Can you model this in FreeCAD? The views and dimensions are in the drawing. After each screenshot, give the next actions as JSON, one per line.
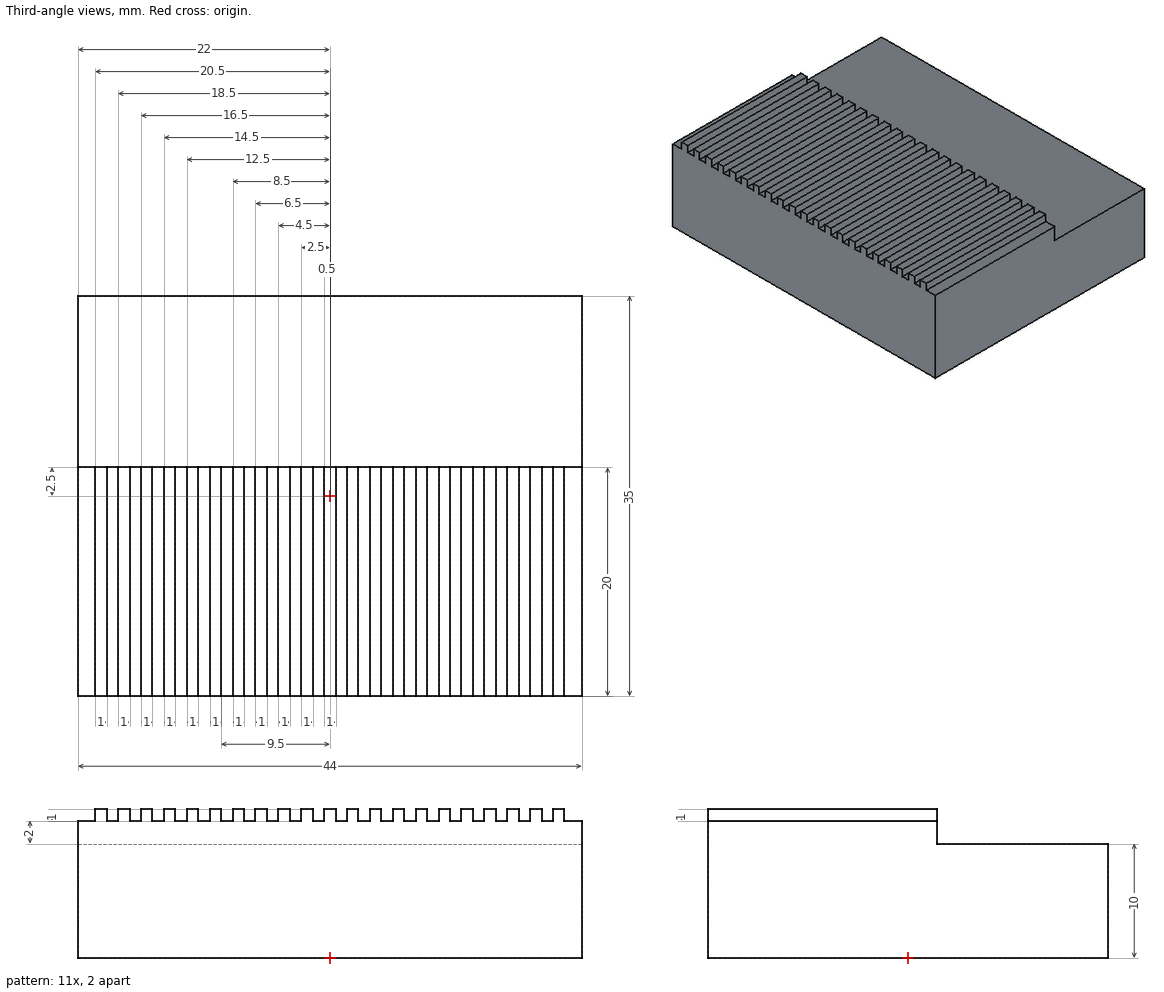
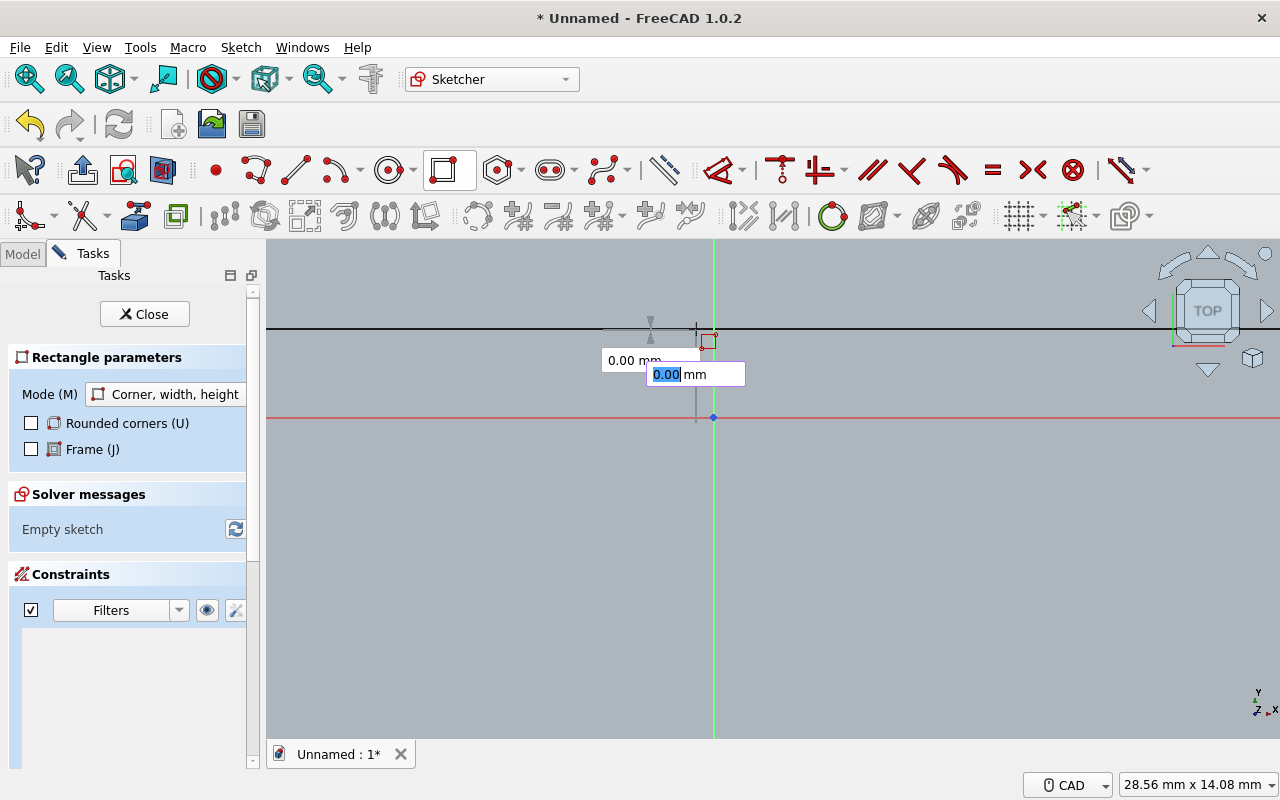
{"action": "scroll", "coordinate": [697, 330], "scroll_direction": "down", "scroll_amount": 4}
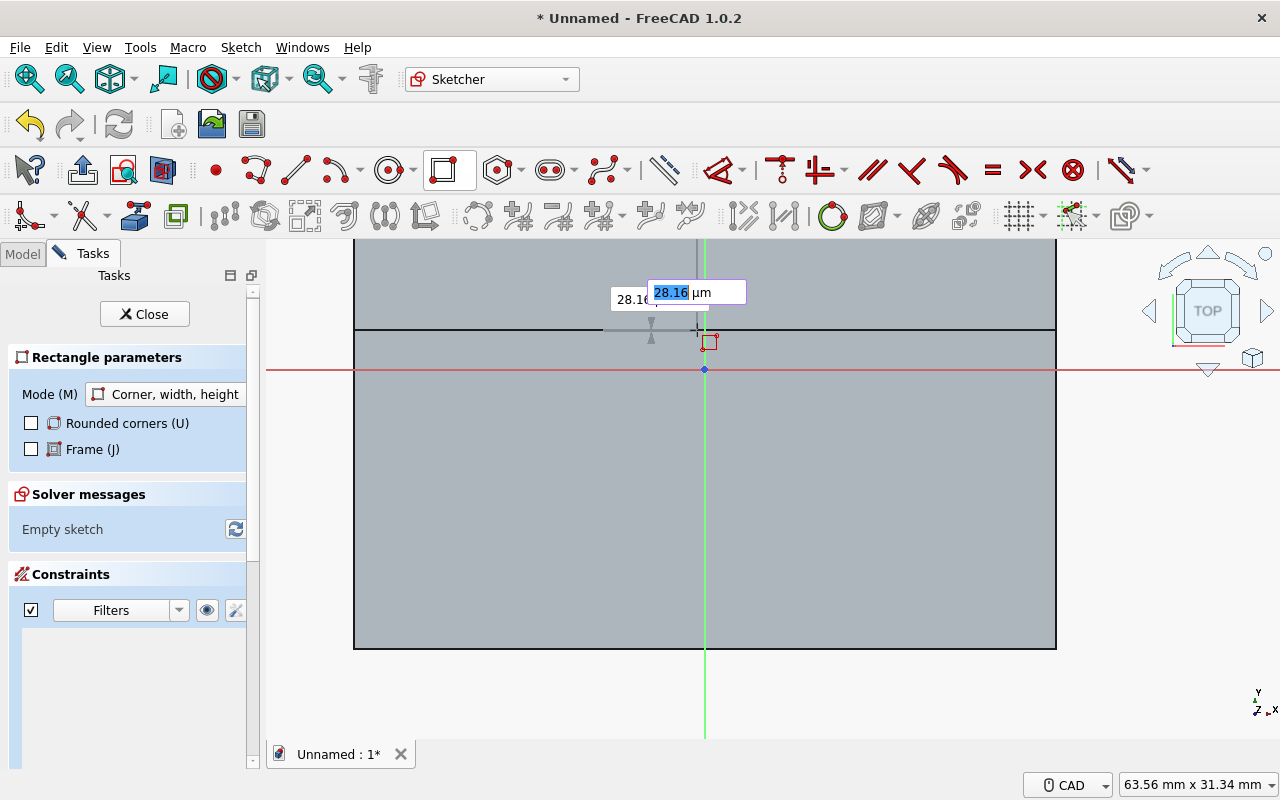
{"action": "scroll", "coordinate": [713, 649], "scroll_direction": "up", "scroll_amount": 4}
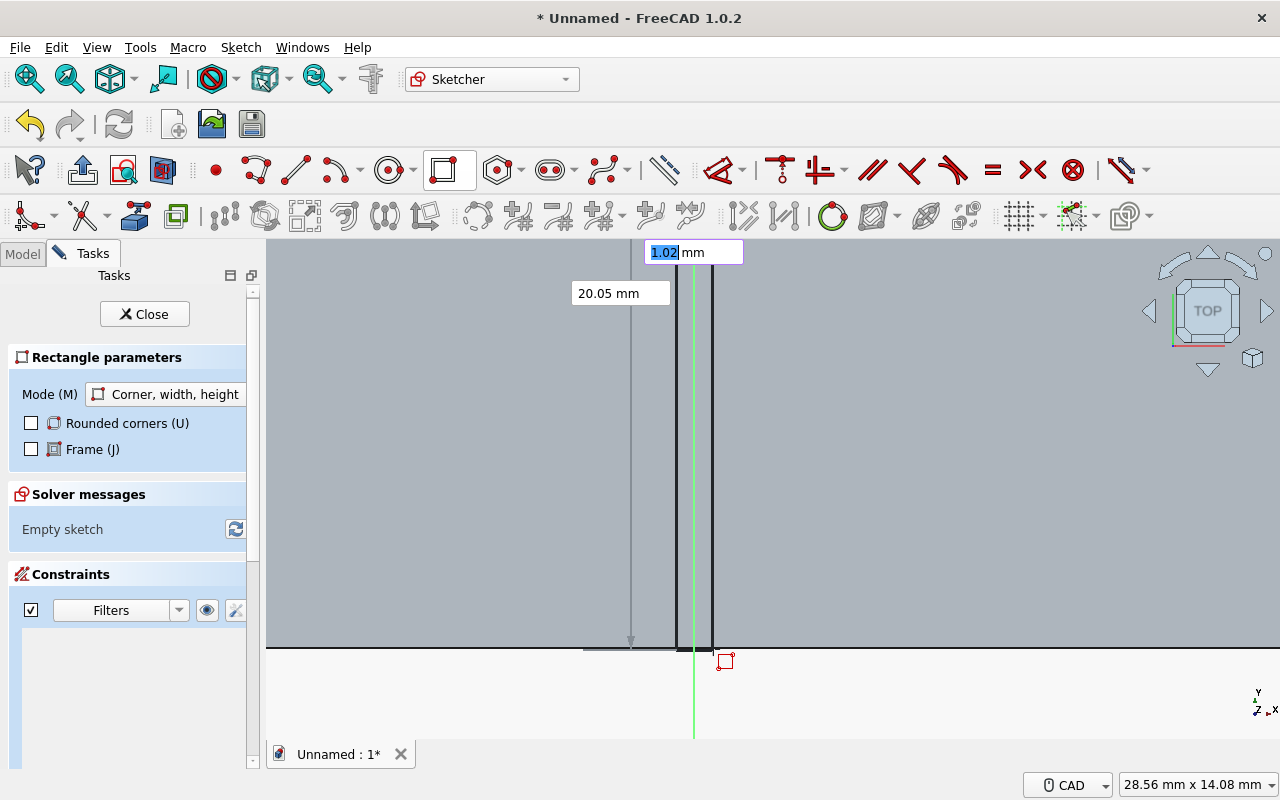
{"action": "left_click", "coordinate": [712, 648]}
{"action": "key", "text": "Escape"}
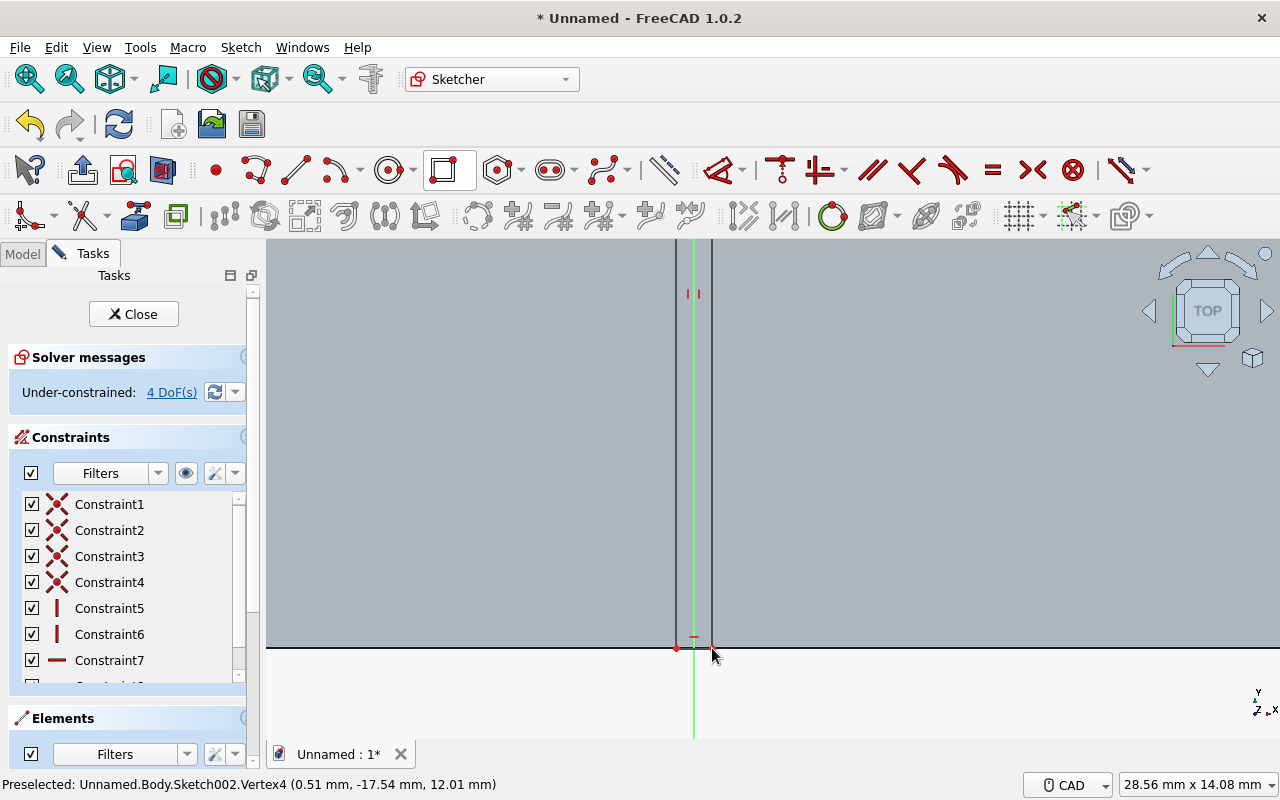
{"action": "left_click", "coordinate": [691, 649]}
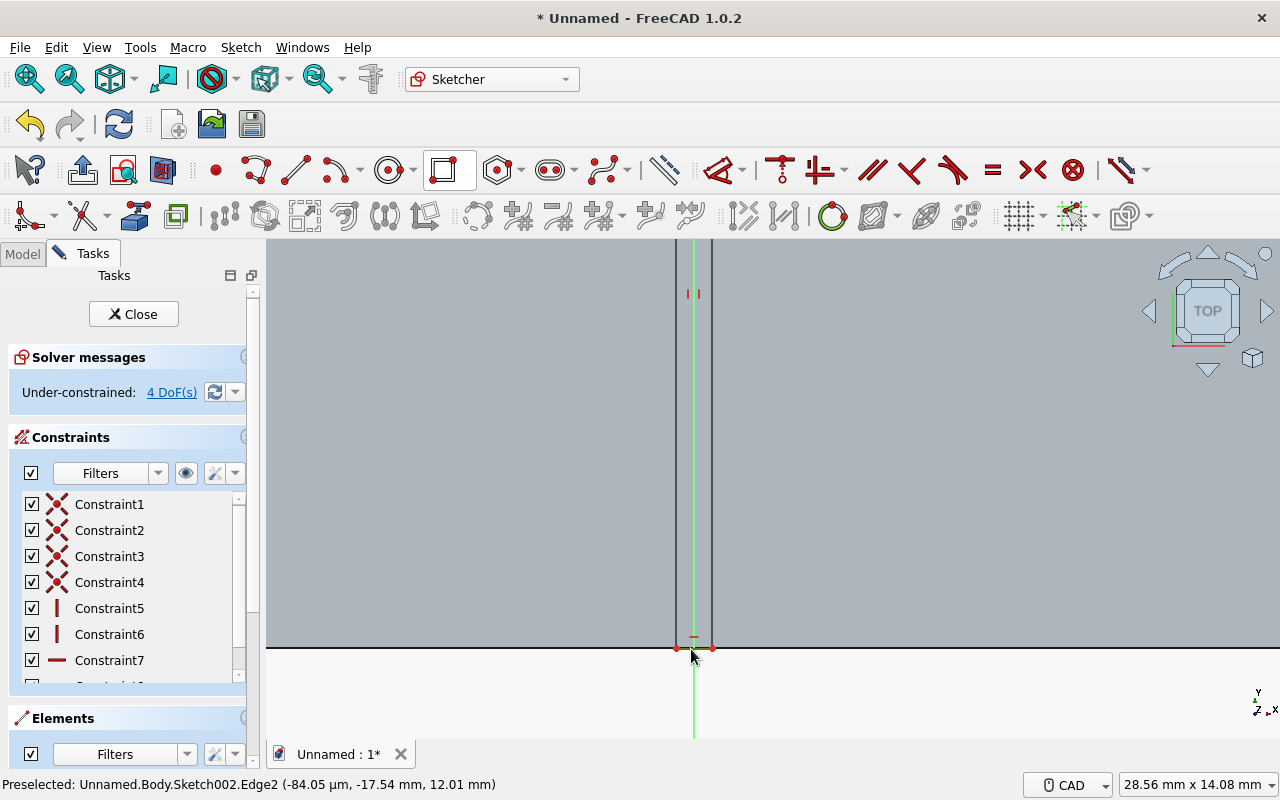
{"action": "left_click", "coordinate": [744, 170]}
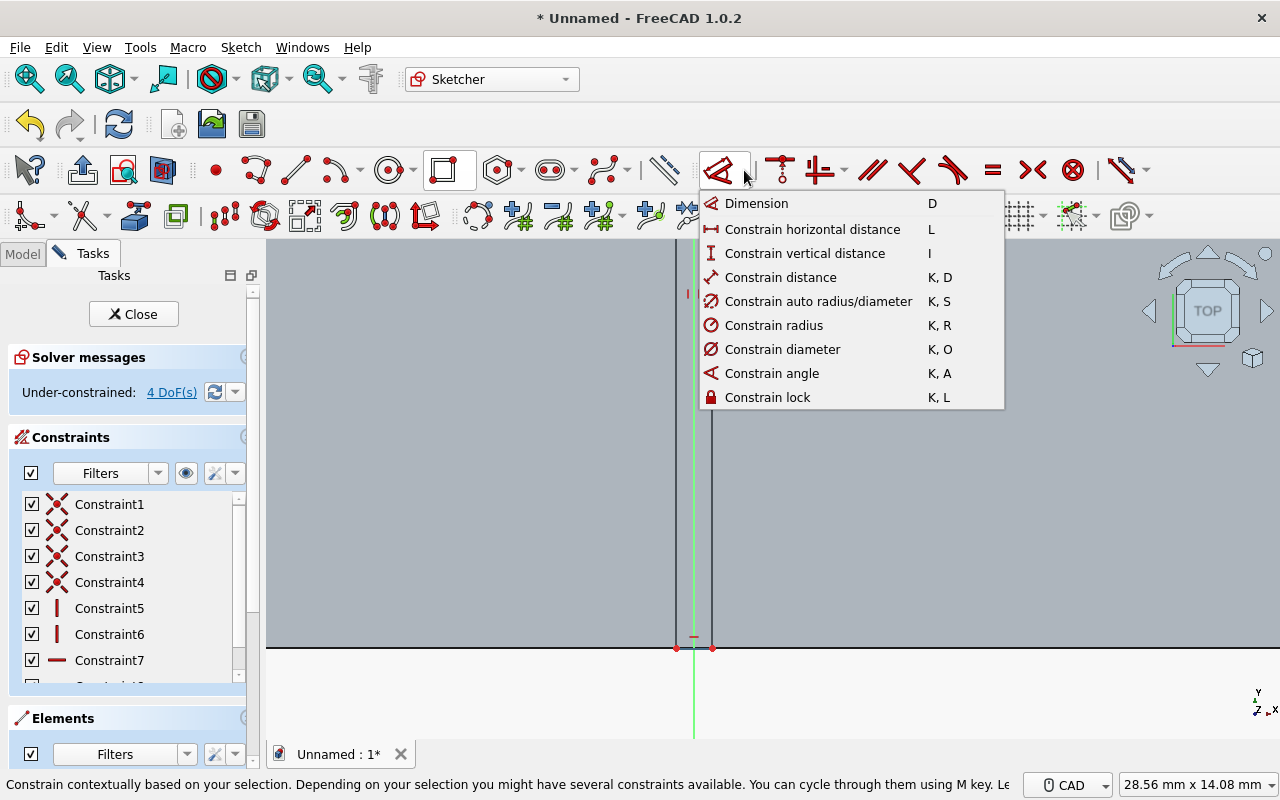
{"action": "left_click", "coordinate": [852, 229]}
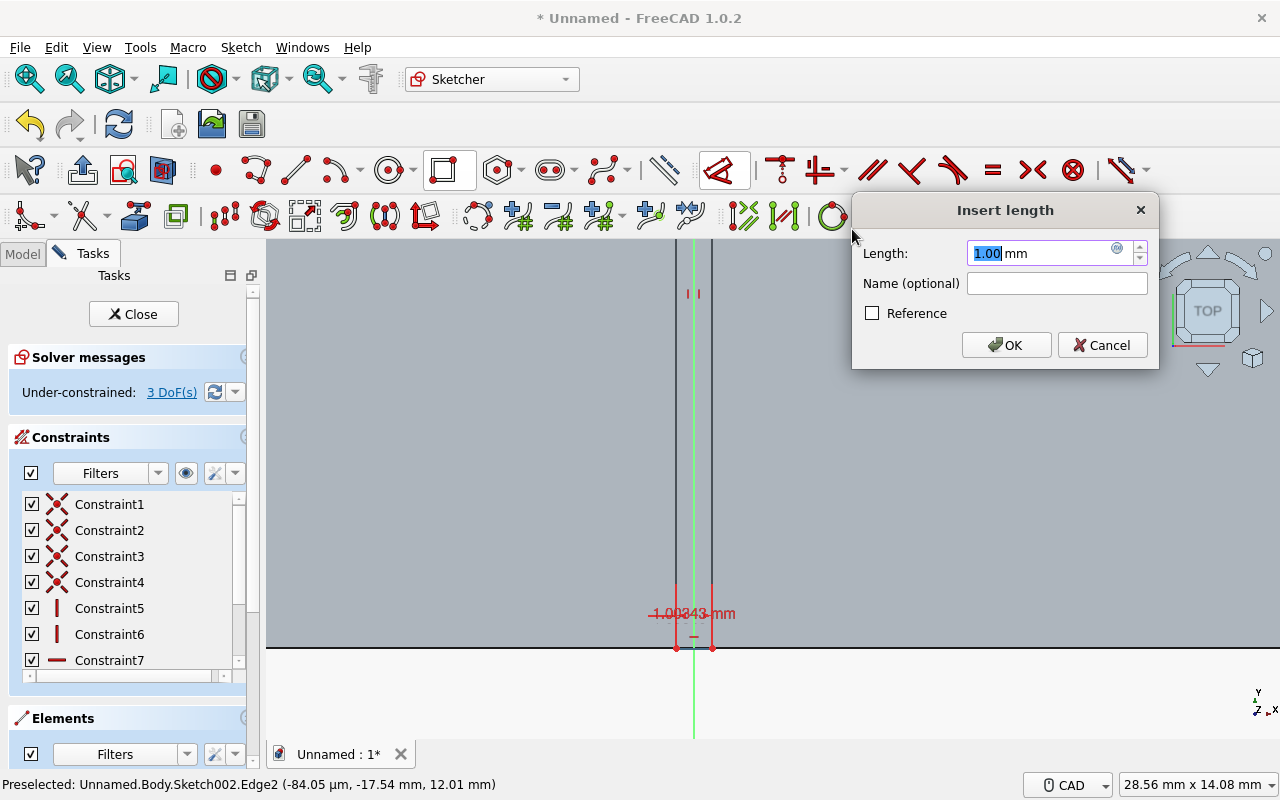
{"action": "type", "text": "1"}
{"action": "key", "text": "Return"}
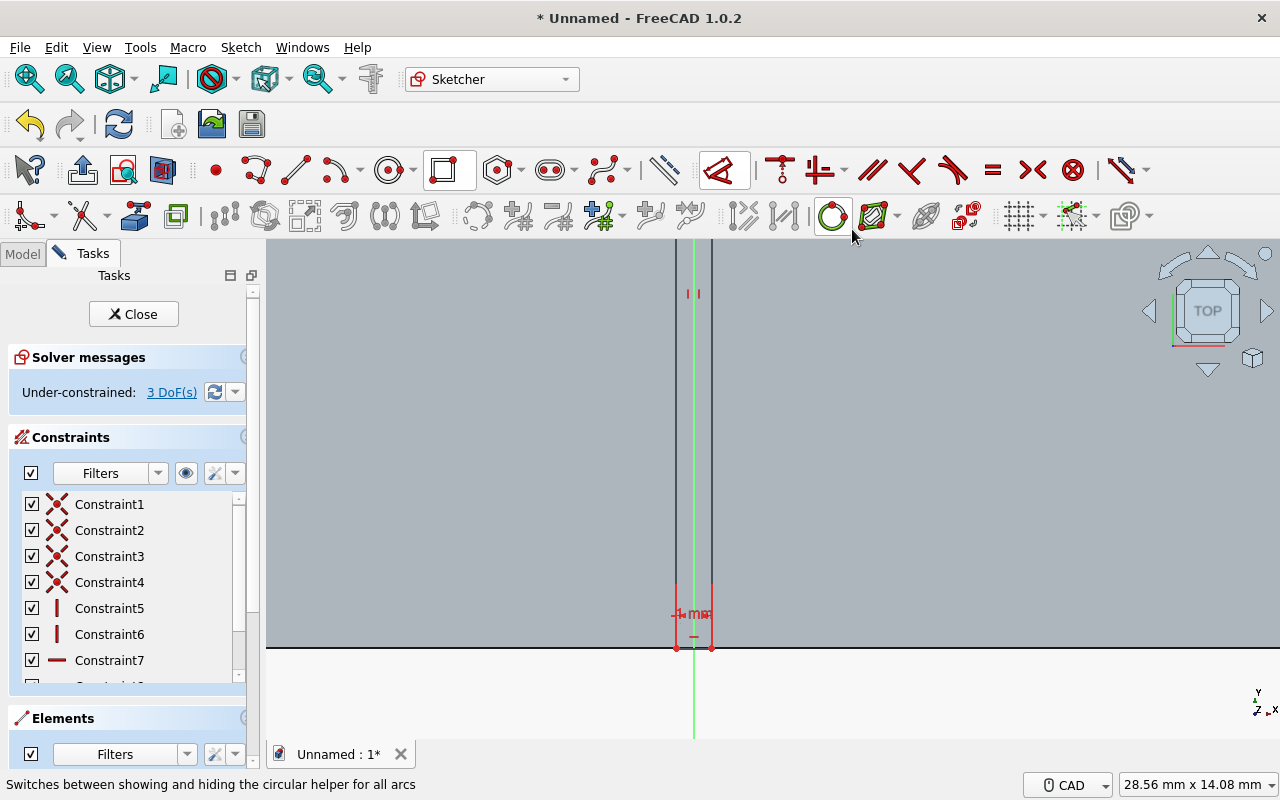
{"action": "left_click", "coordinate": [676, 436]}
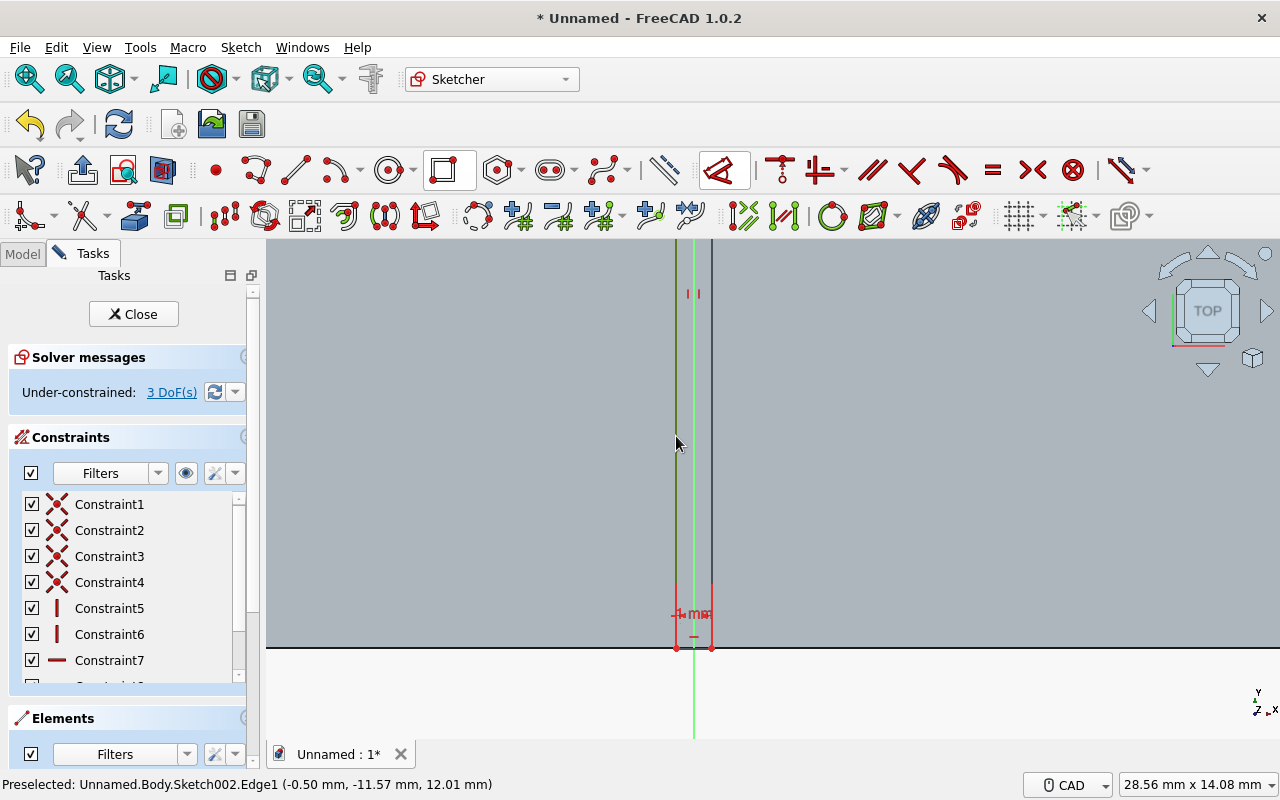
{"action": "key", "text": "i"}